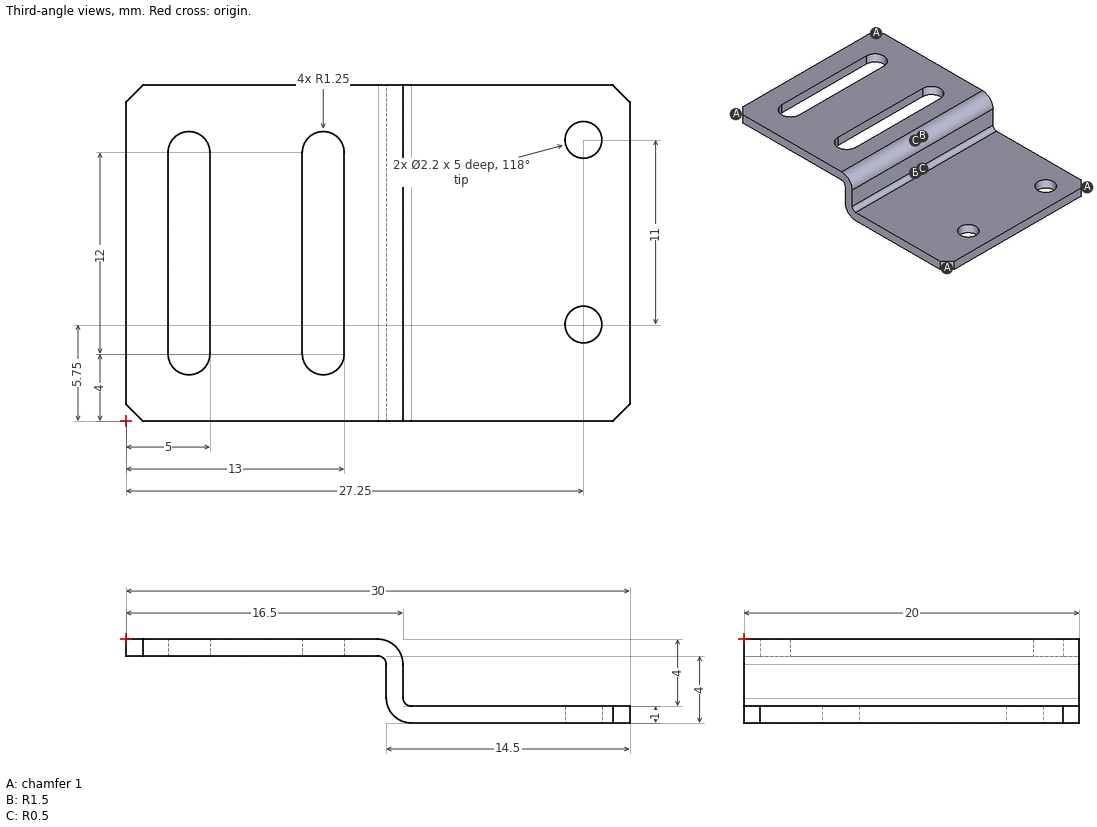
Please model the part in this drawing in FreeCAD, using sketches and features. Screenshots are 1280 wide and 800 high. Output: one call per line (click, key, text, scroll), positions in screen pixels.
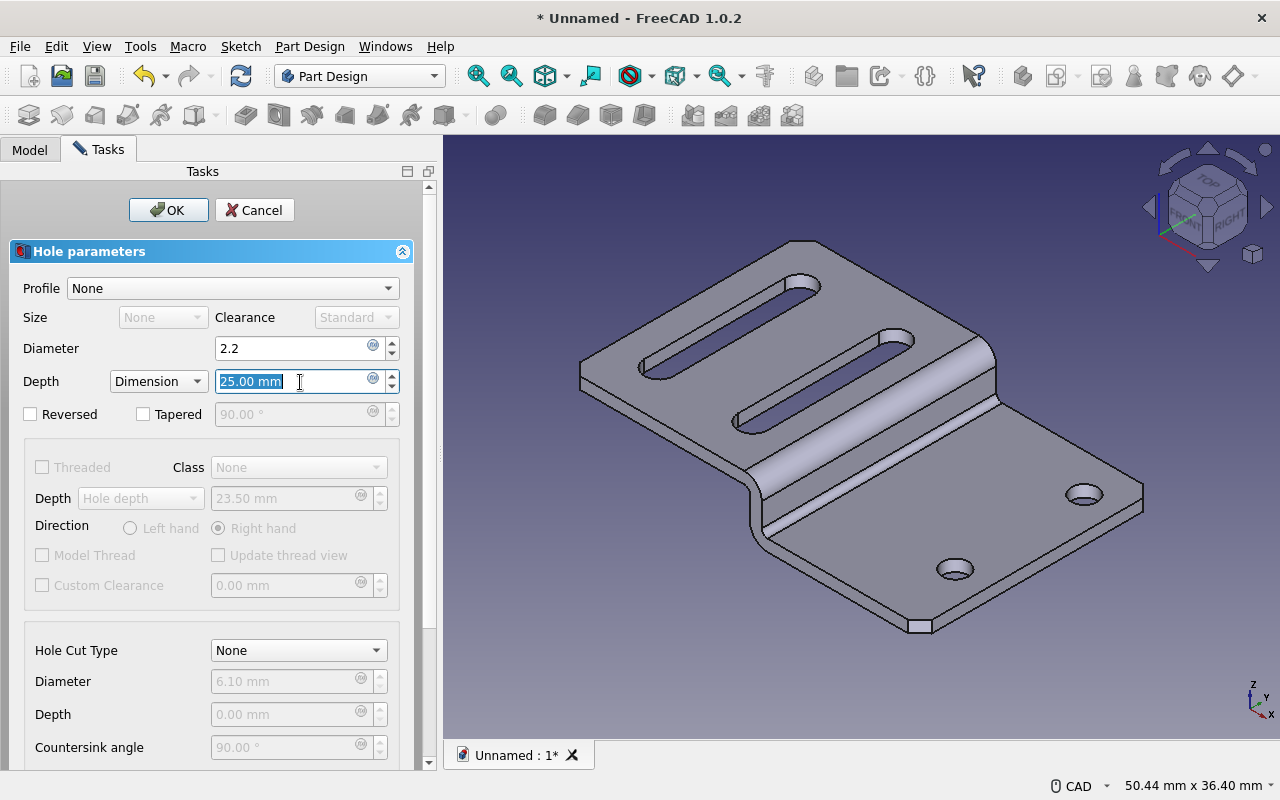
text(5)
key(Tab)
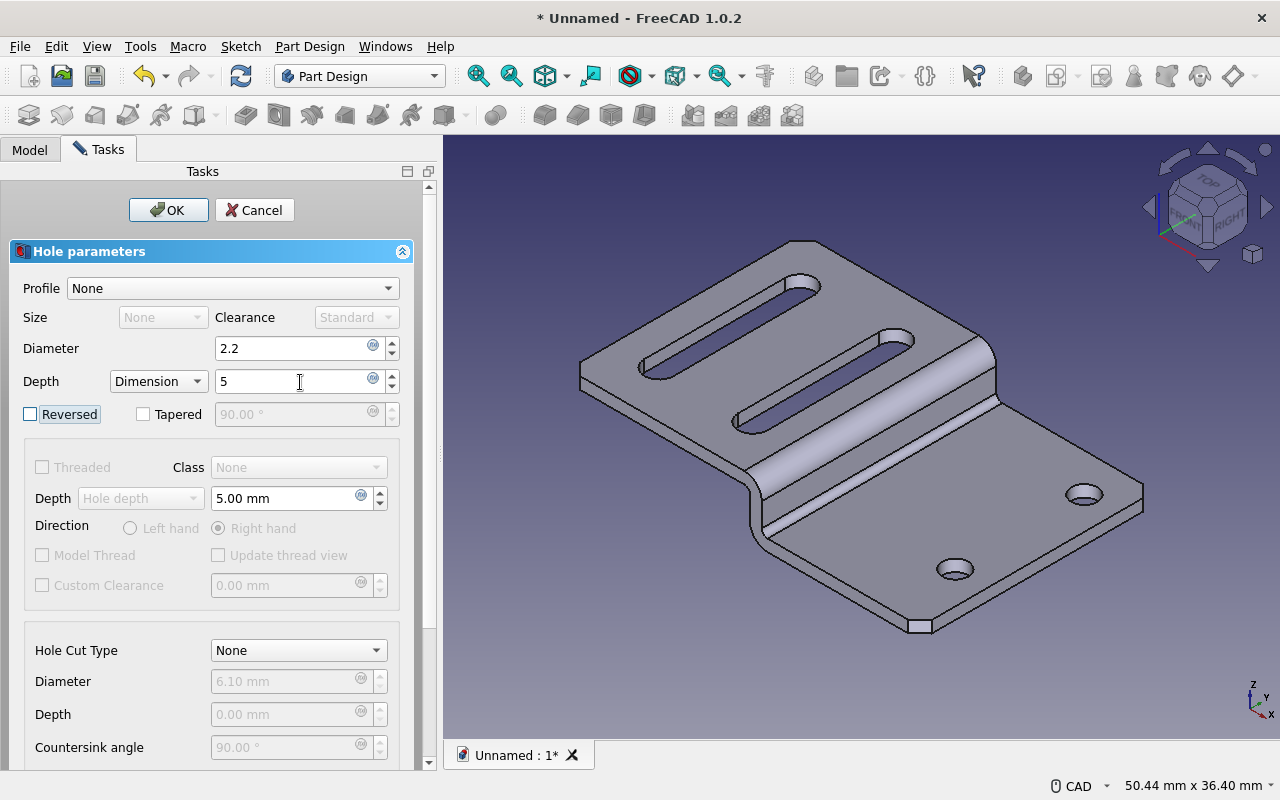
click(169, 210)